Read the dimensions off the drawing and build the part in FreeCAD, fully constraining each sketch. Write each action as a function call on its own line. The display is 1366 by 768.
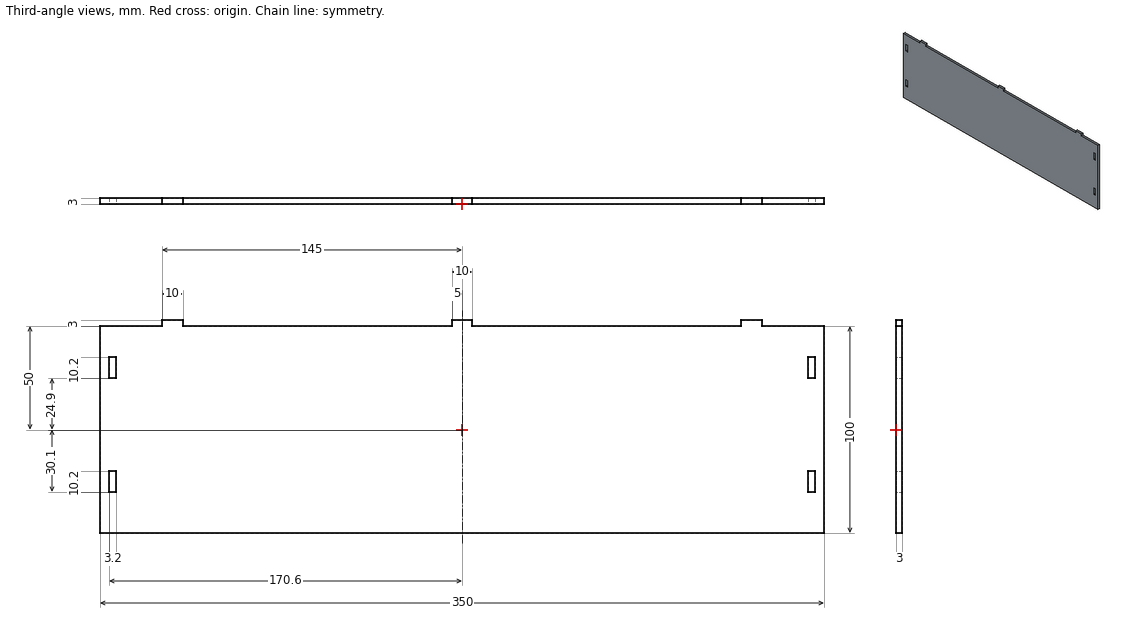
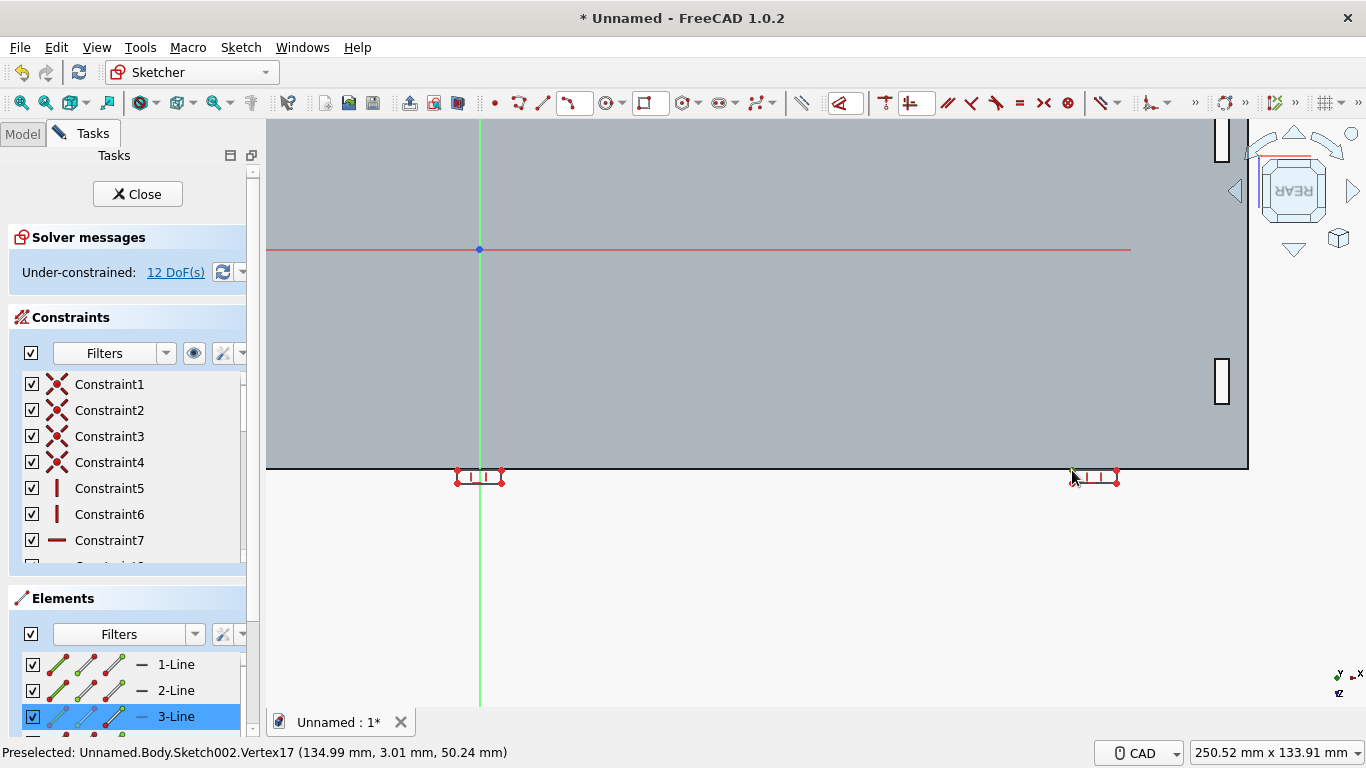
click(480, 641)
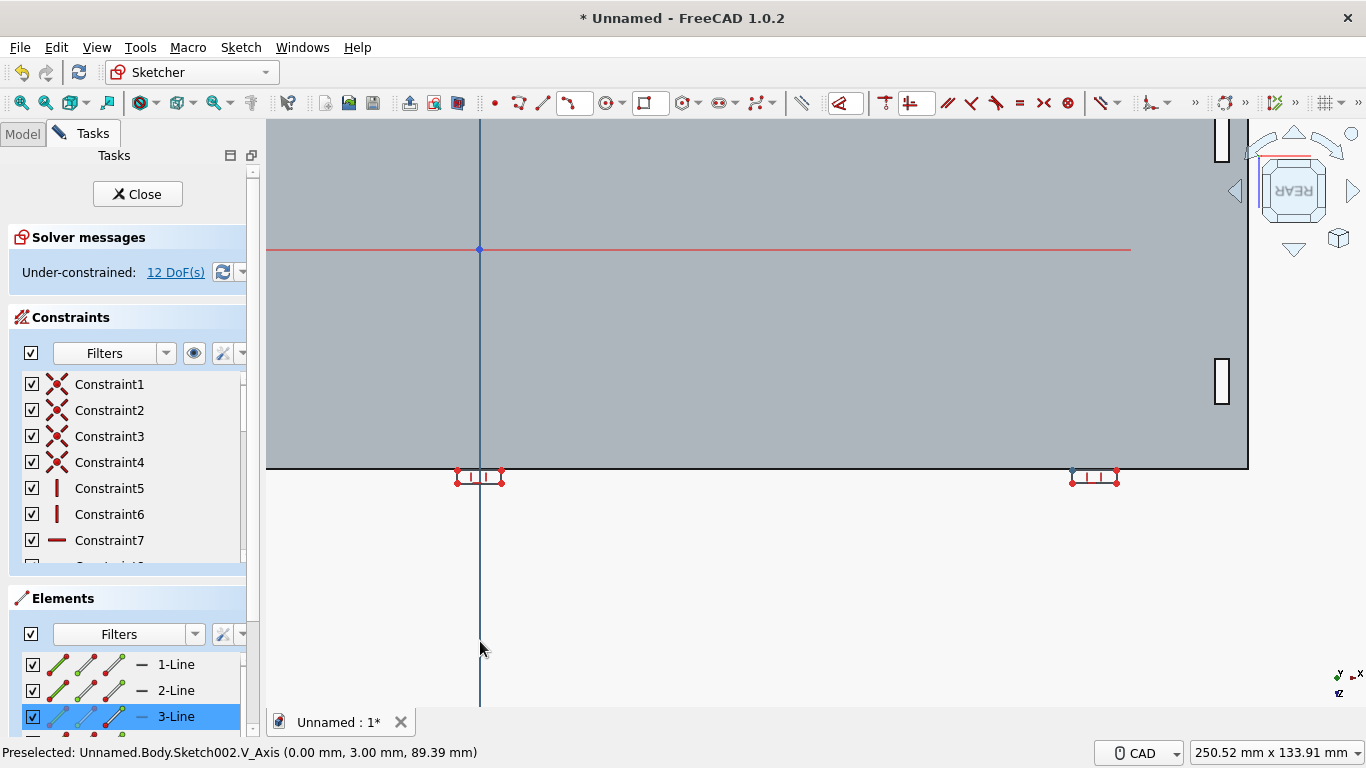
click(1044, 104)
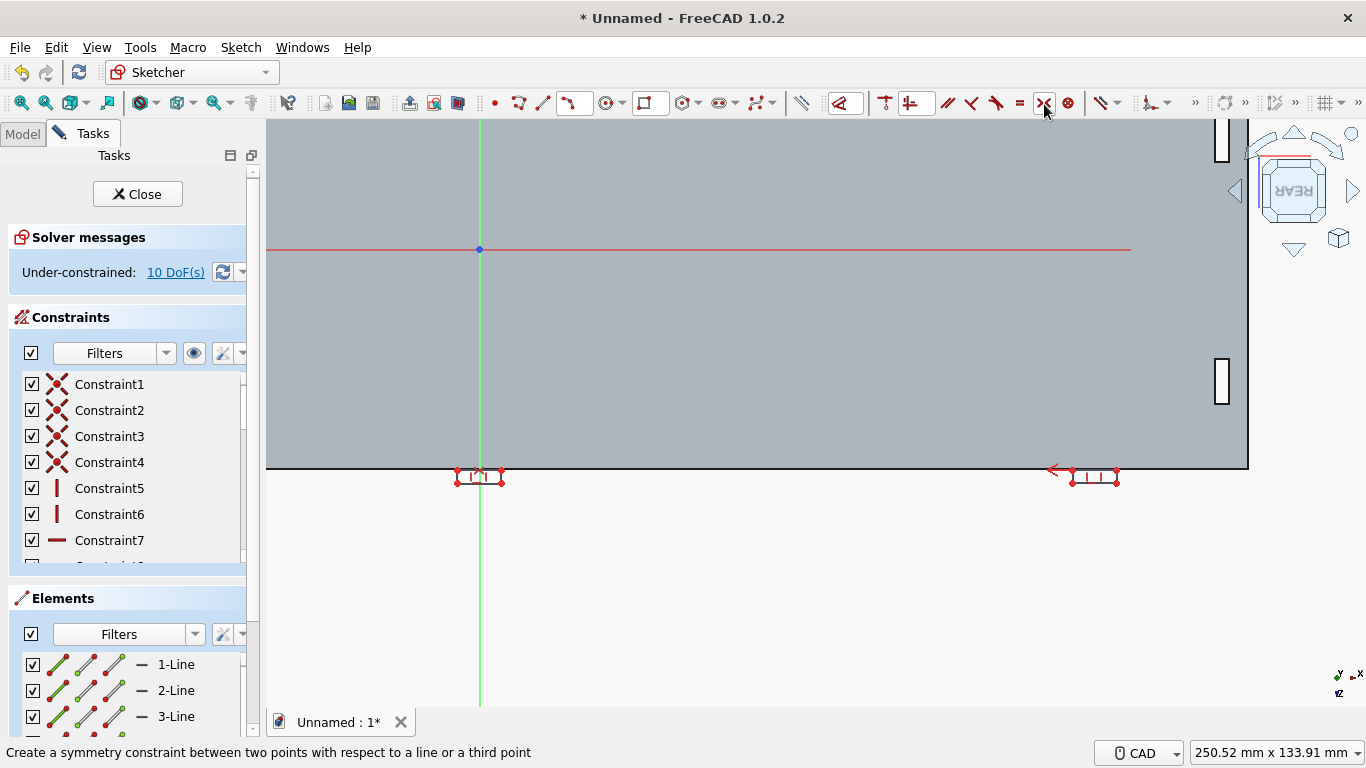
scroll(1073, 470, down, 3)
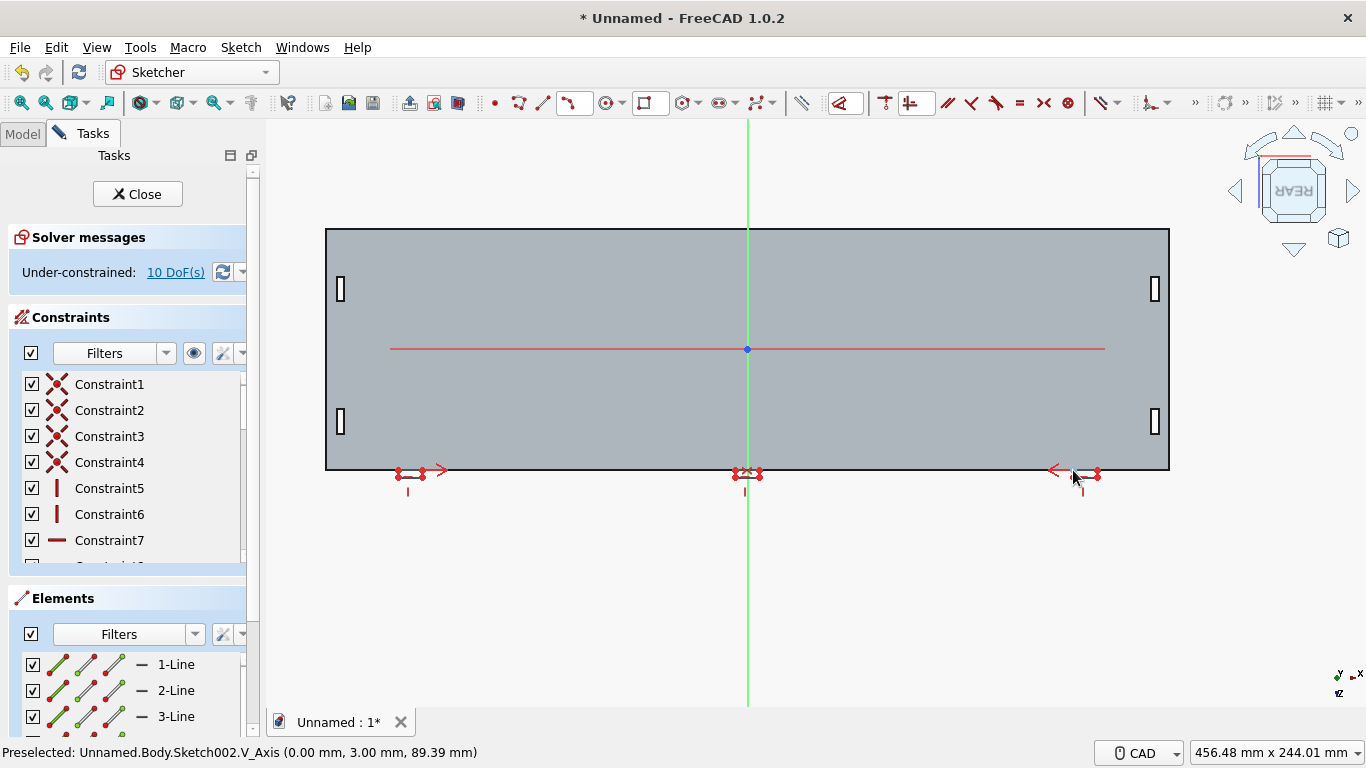
scroll(398, 478, up, 3)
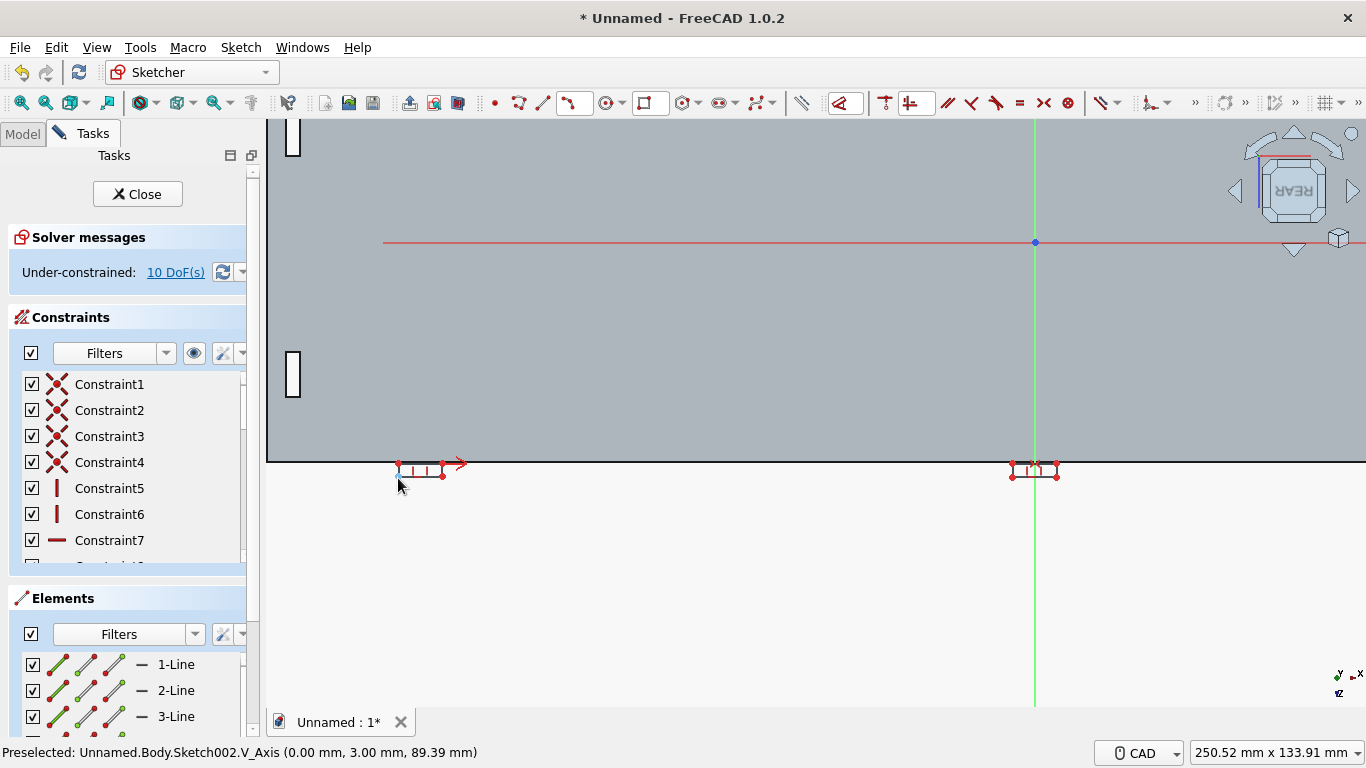
click(399, 477)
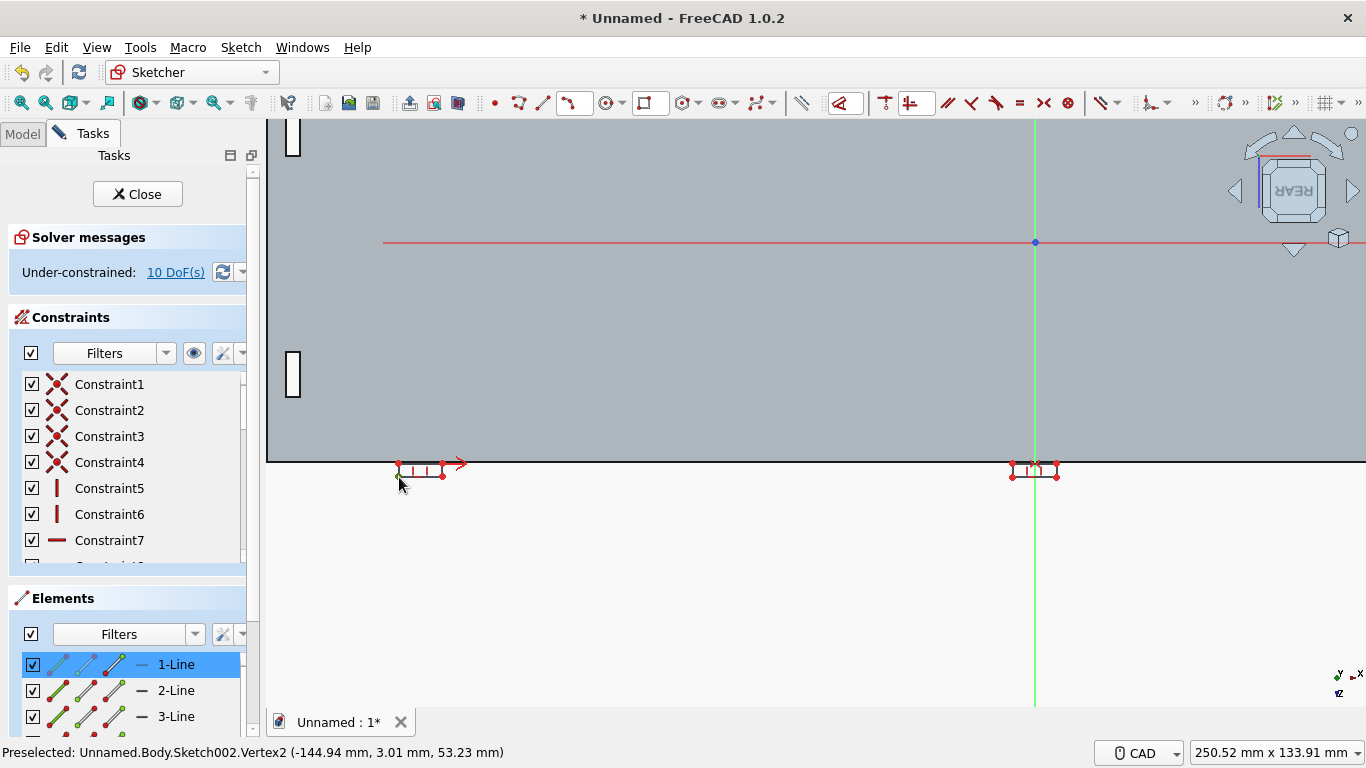
scroll(398, 478, down, 3)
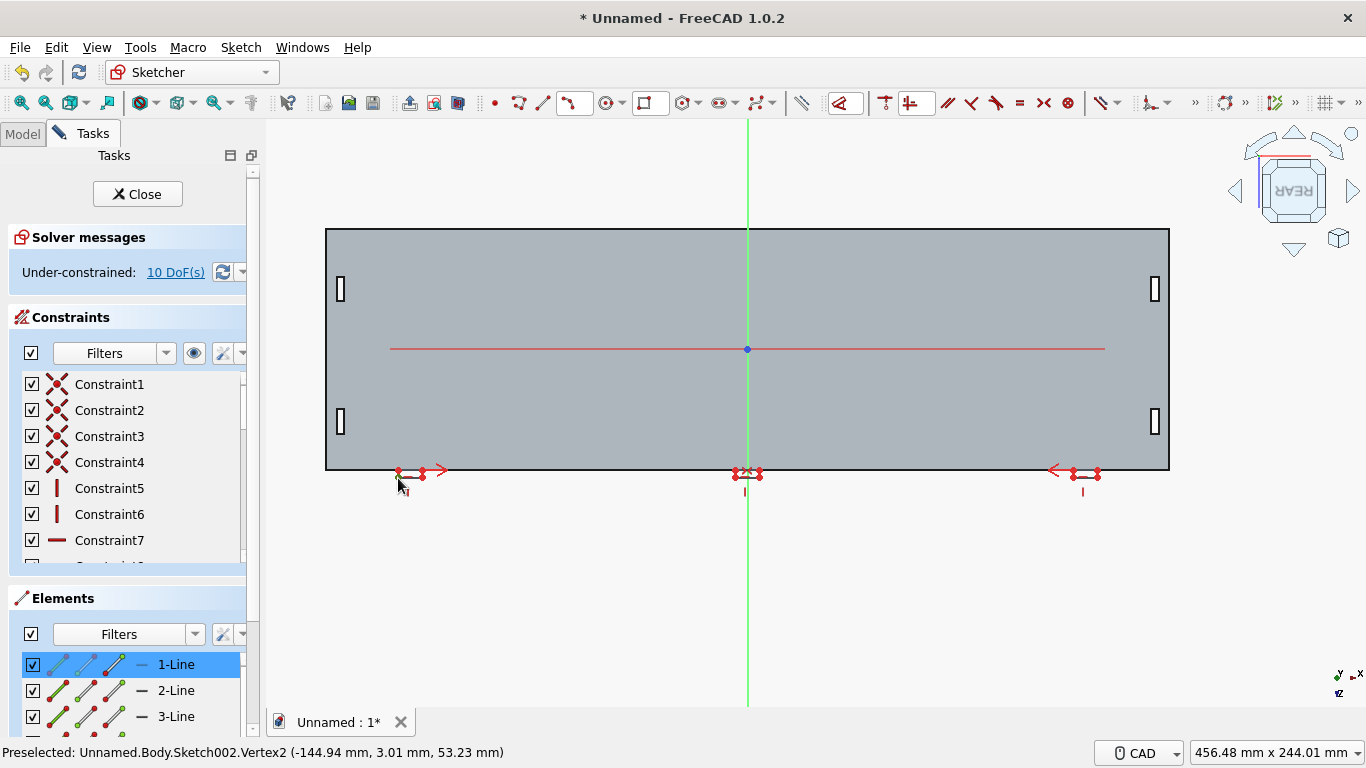
scroll(1097, 478, up, 3)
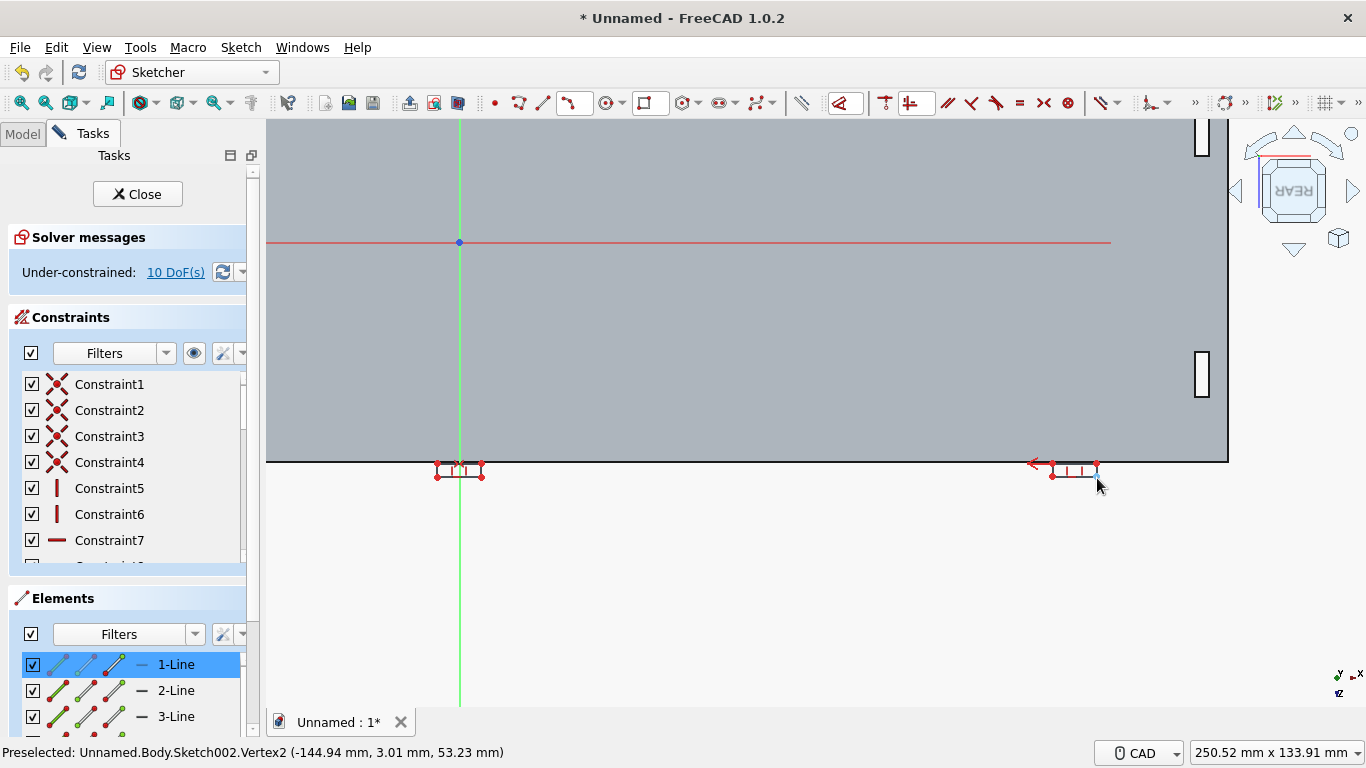
click(1097, 477)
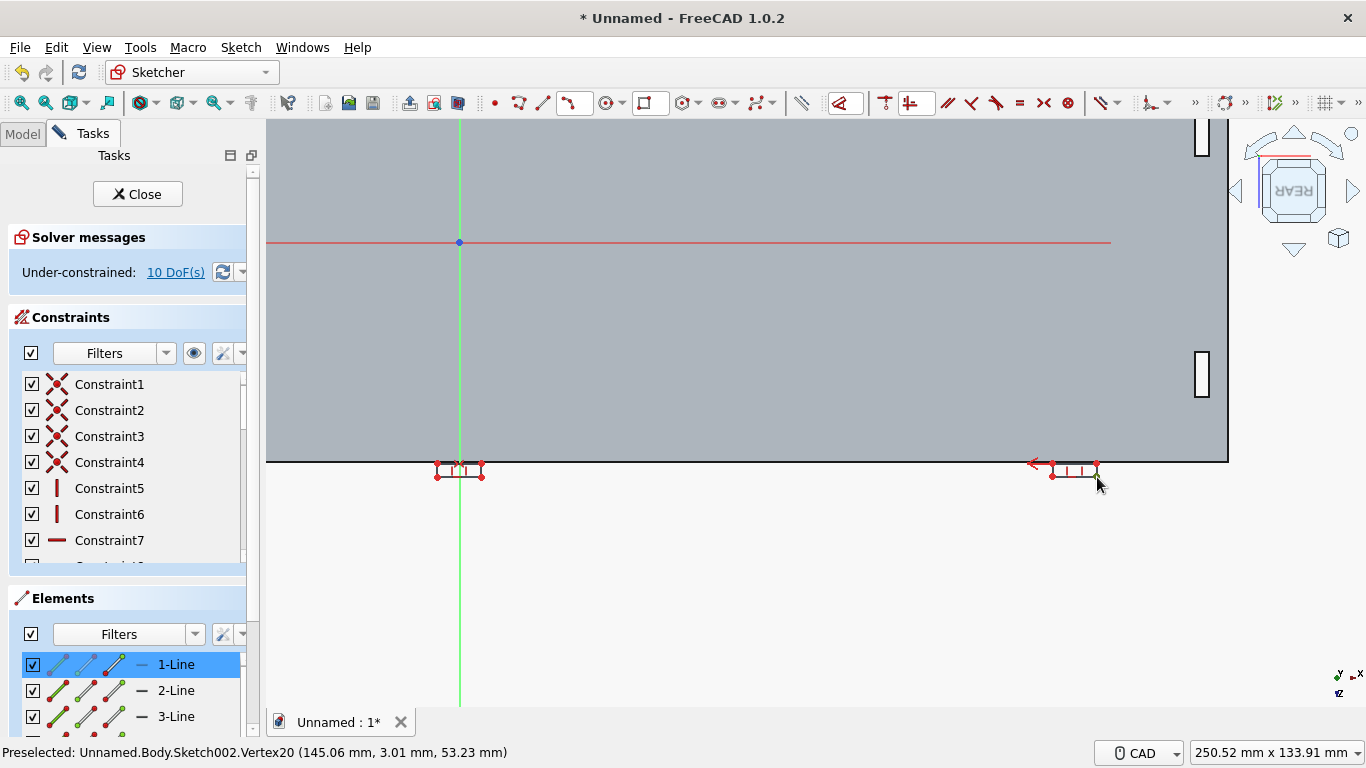
click(460, 641)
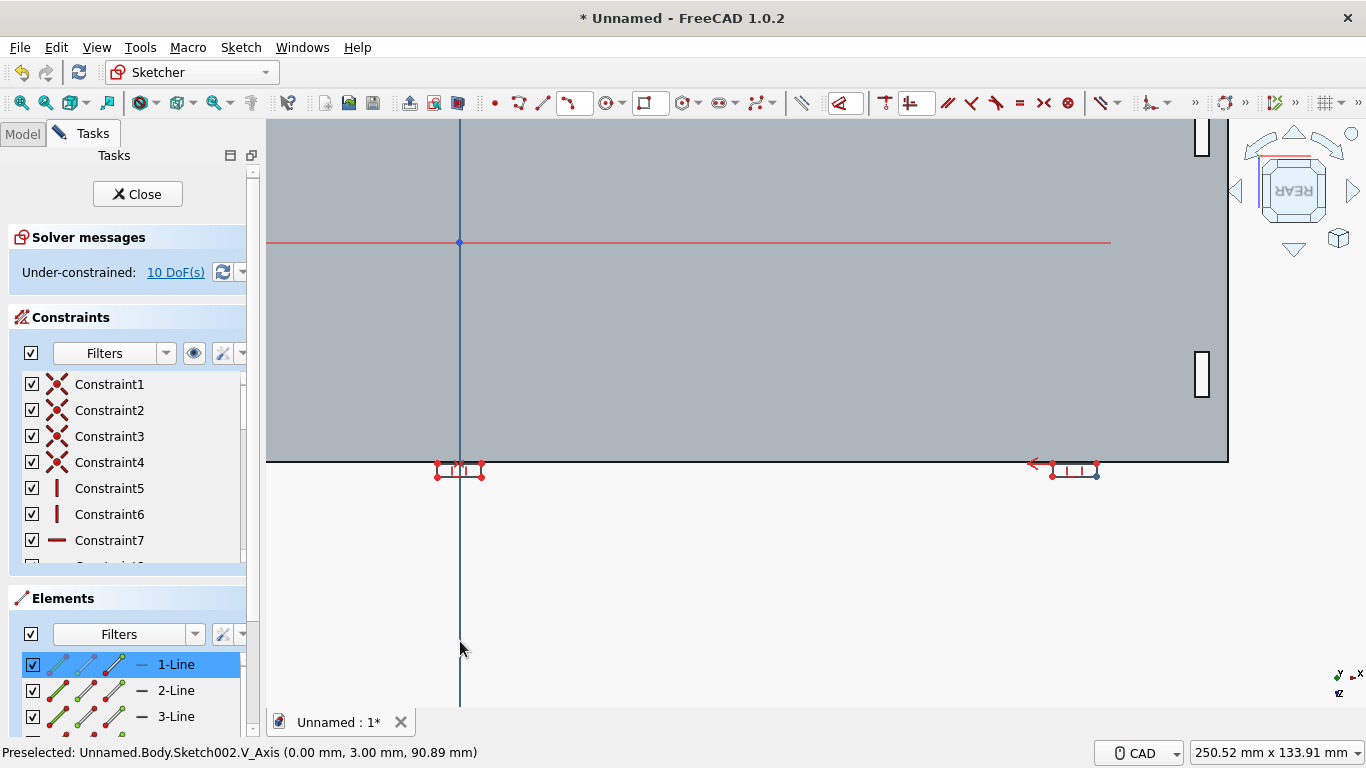
key(s)